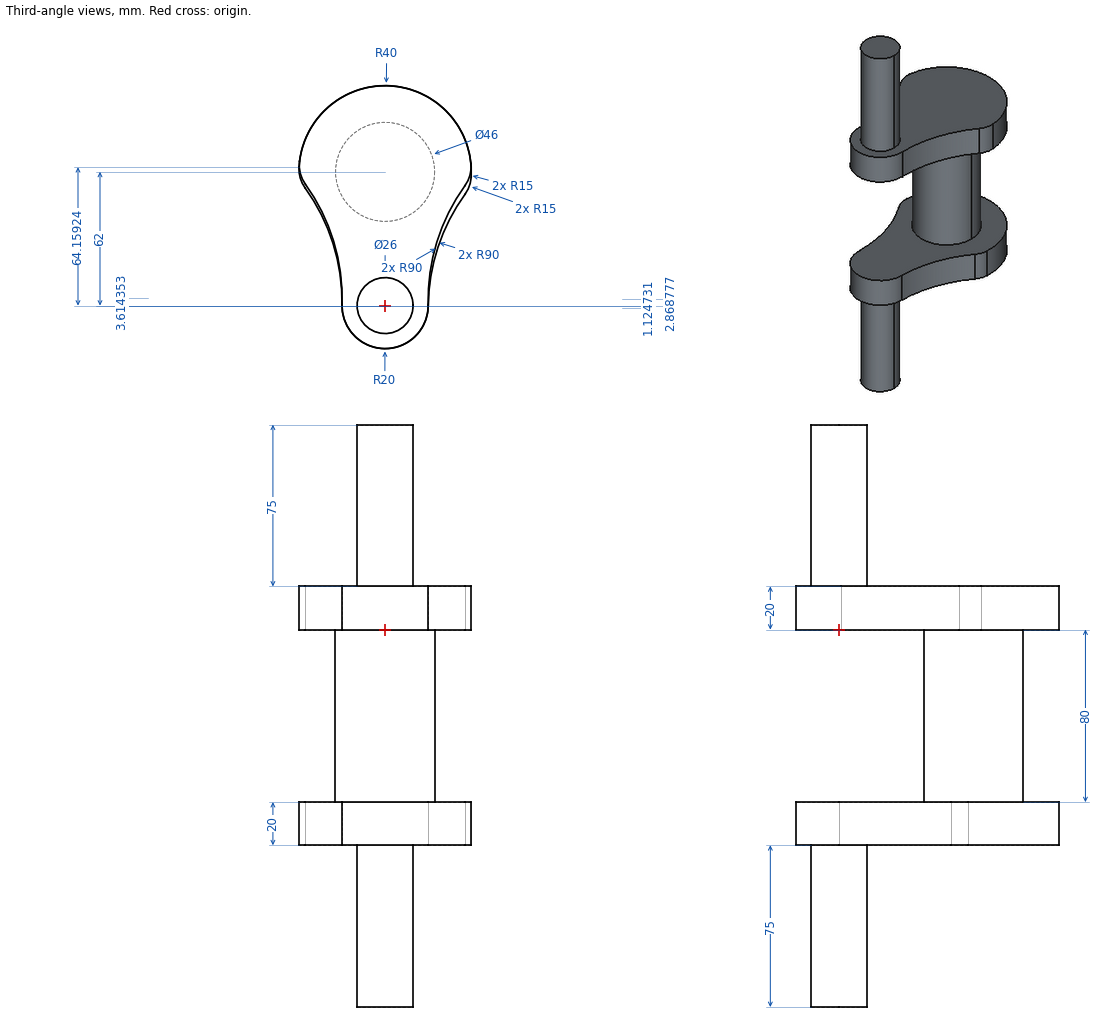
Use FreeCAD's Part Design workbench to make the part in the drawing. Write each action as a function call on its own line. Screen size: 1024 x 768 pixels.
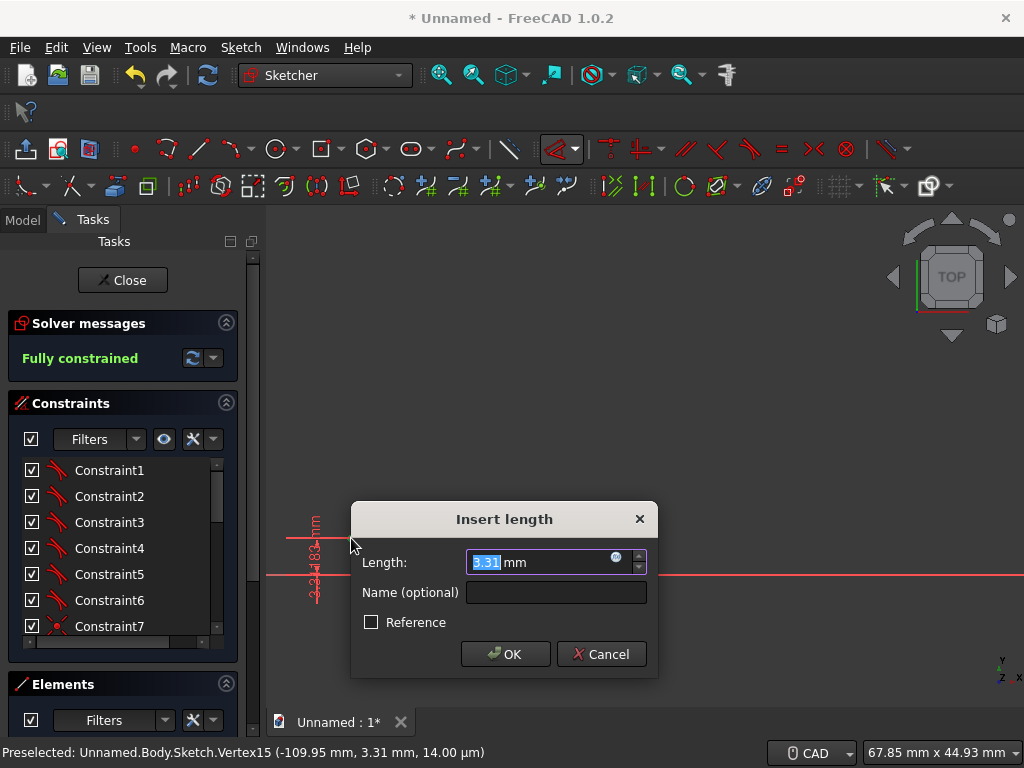
text(3.614353)
key(Return)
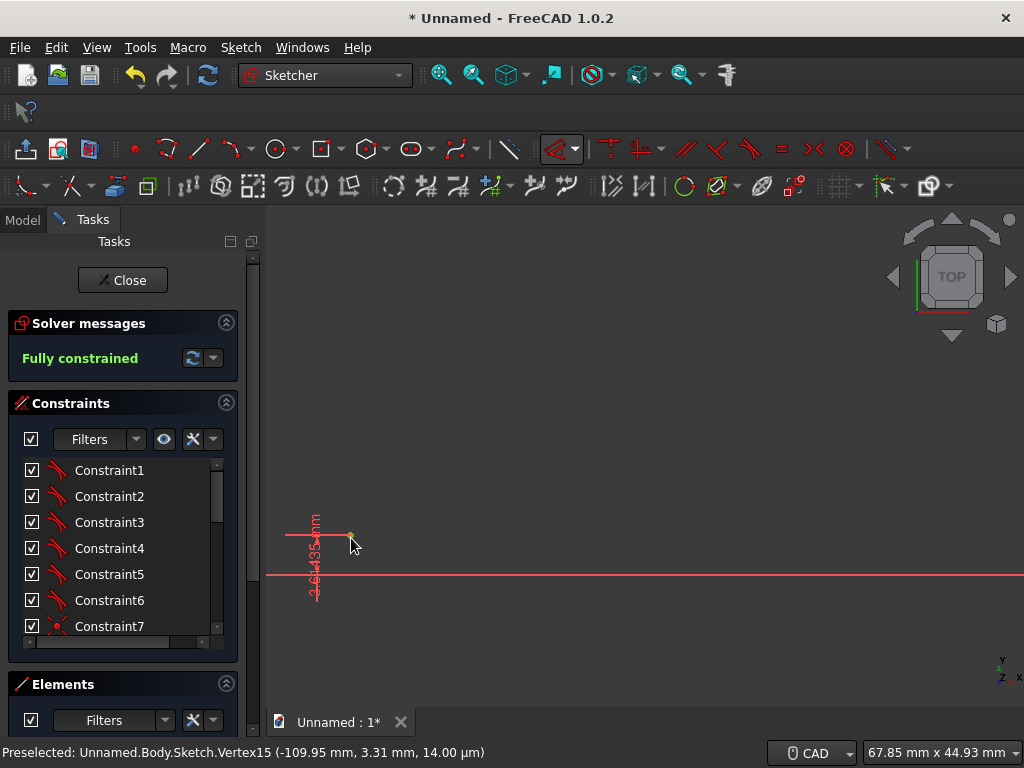
click(123, 280)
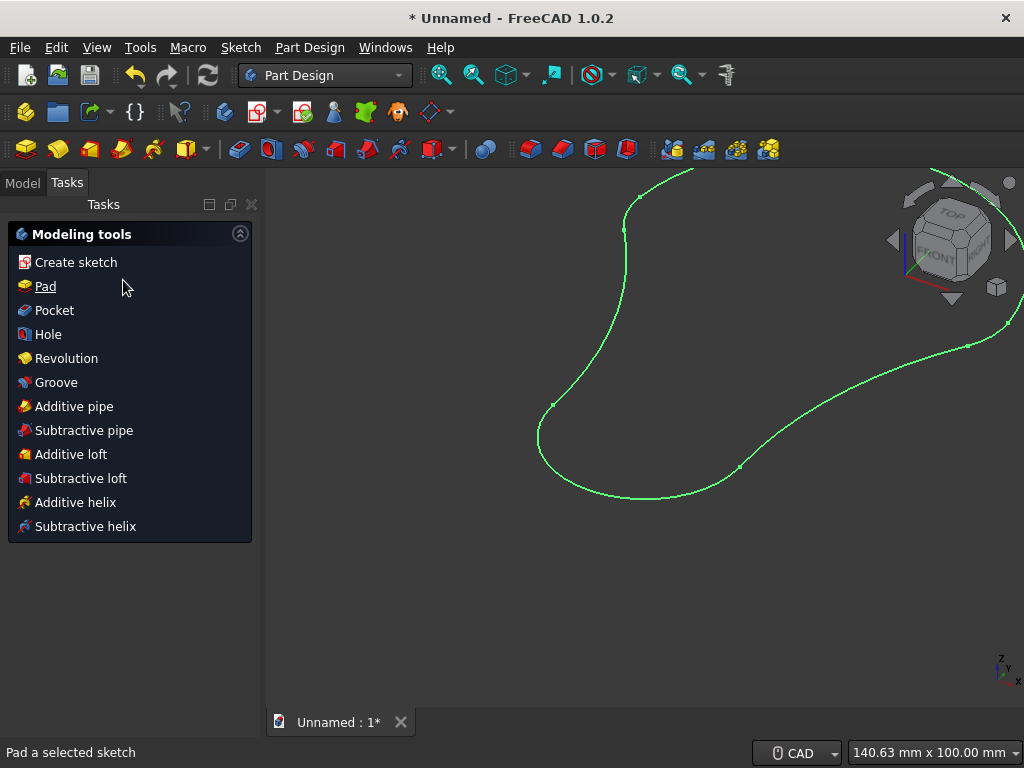
click(26, 150)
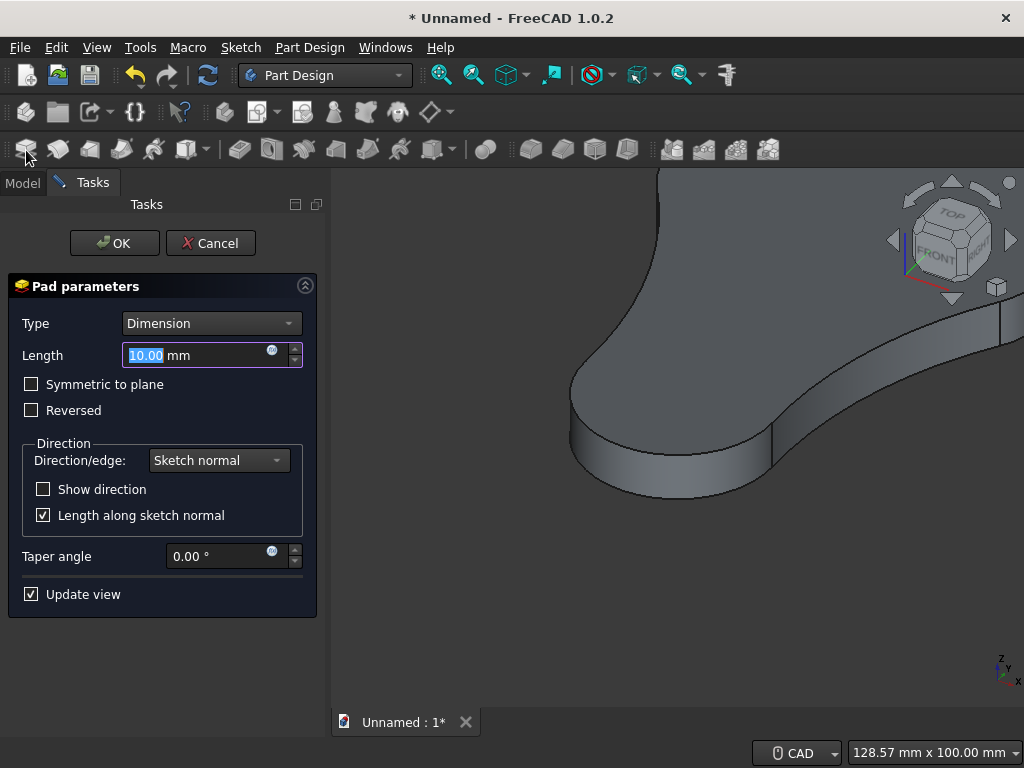
text(20)
key(Tab)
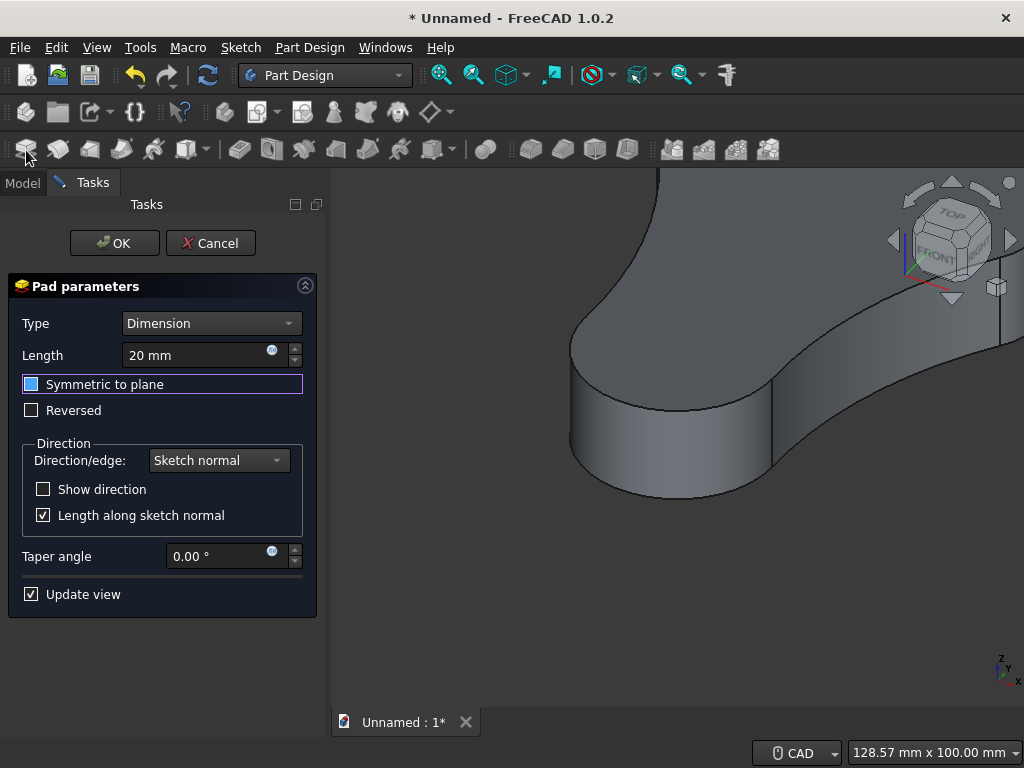
click(115, 243)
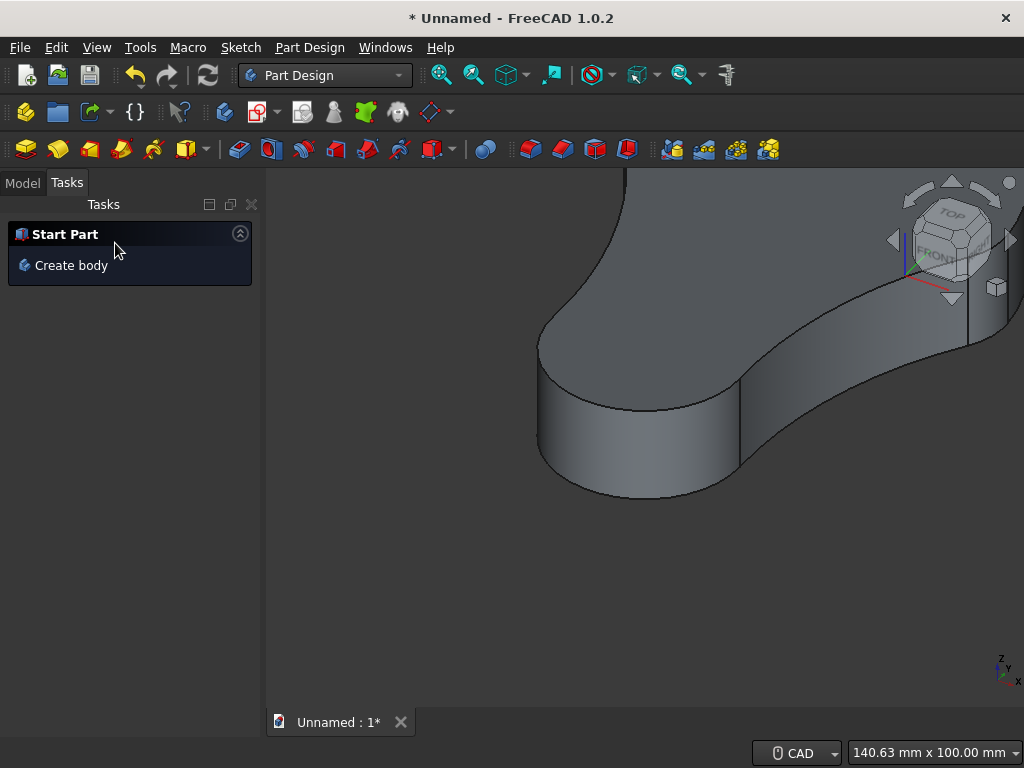
key(v)
key(f)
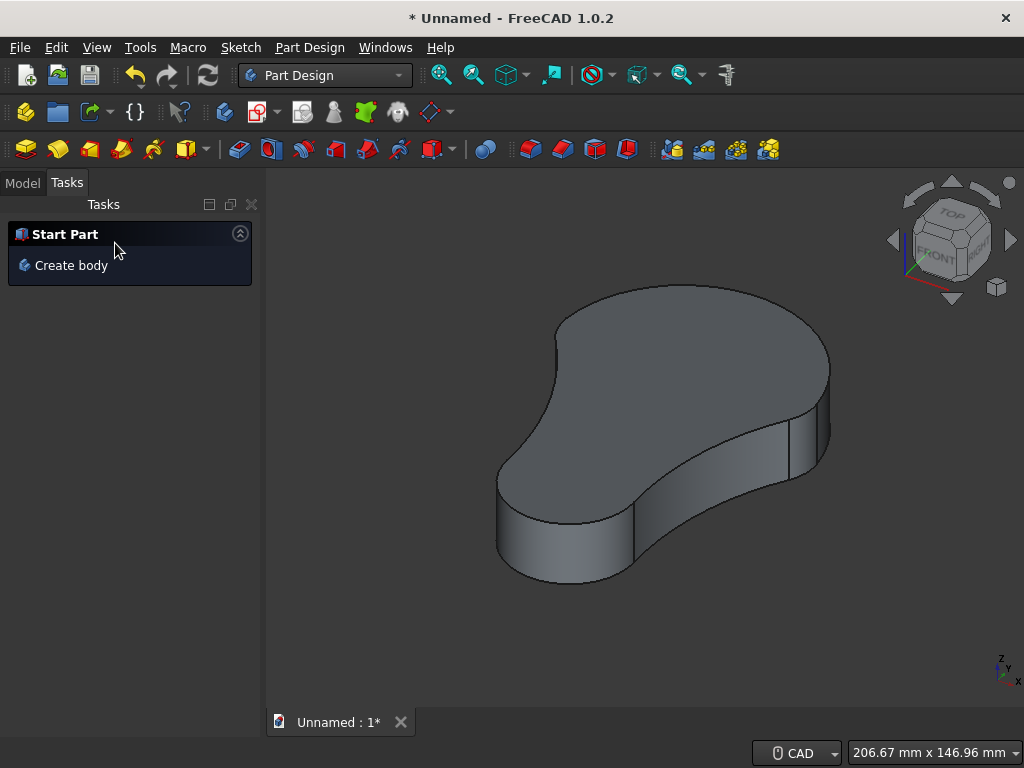
click(677, 375)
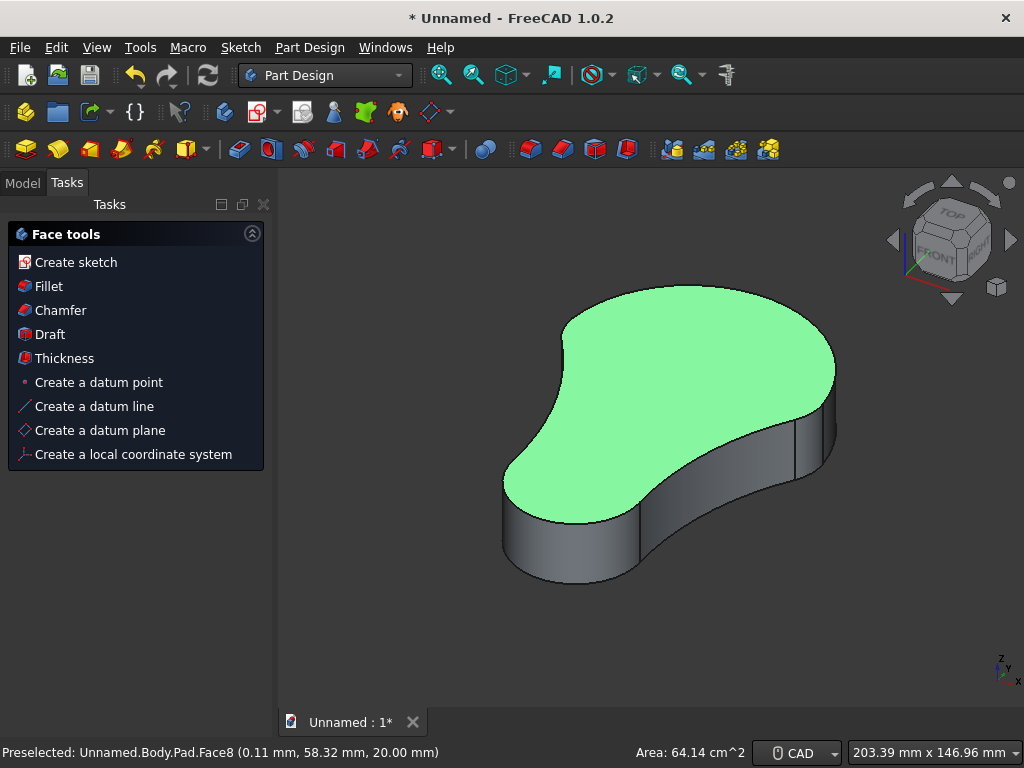
click(258, 112)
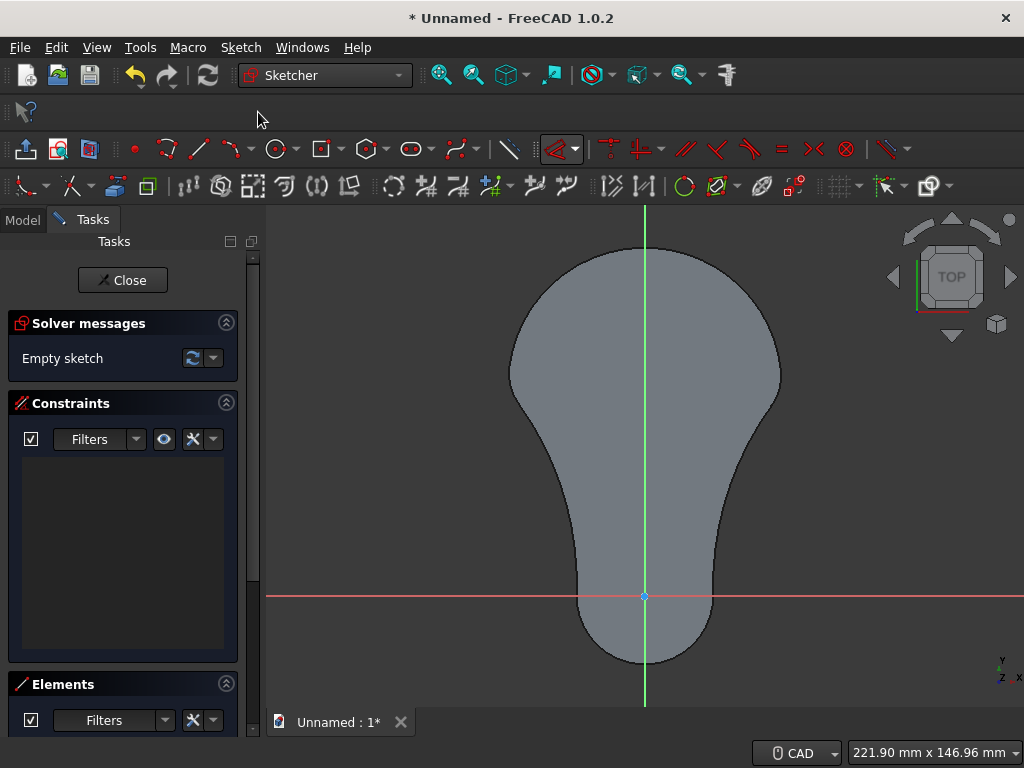
scroll(674, 656, up, 6)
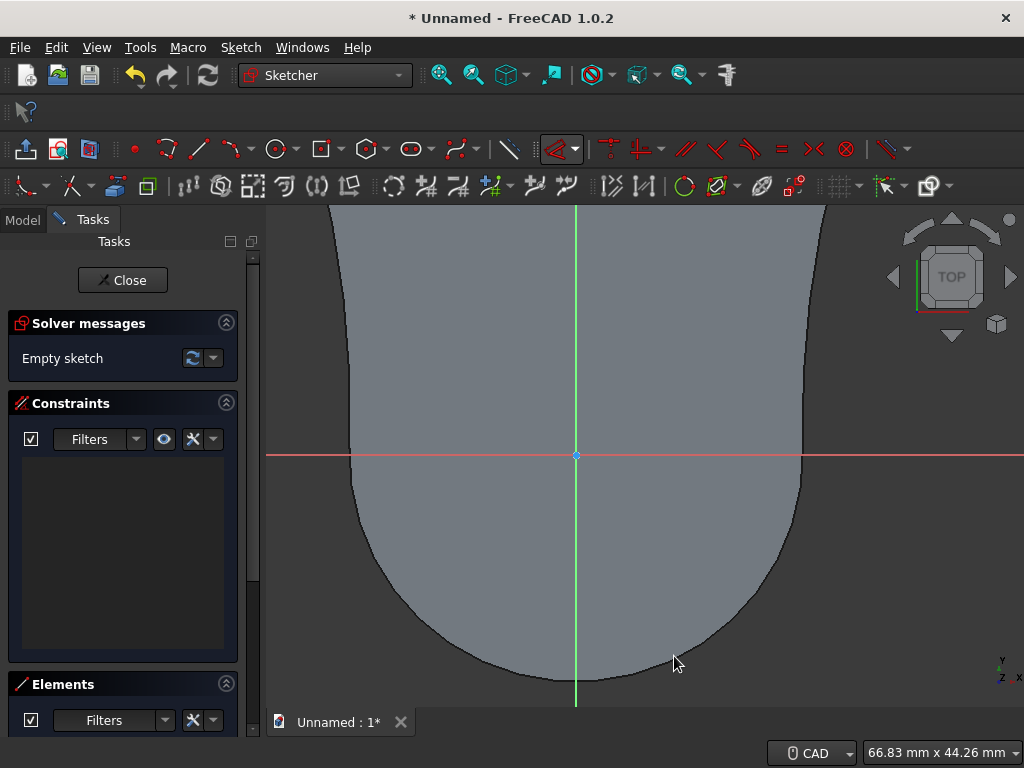
key(g)
key(c)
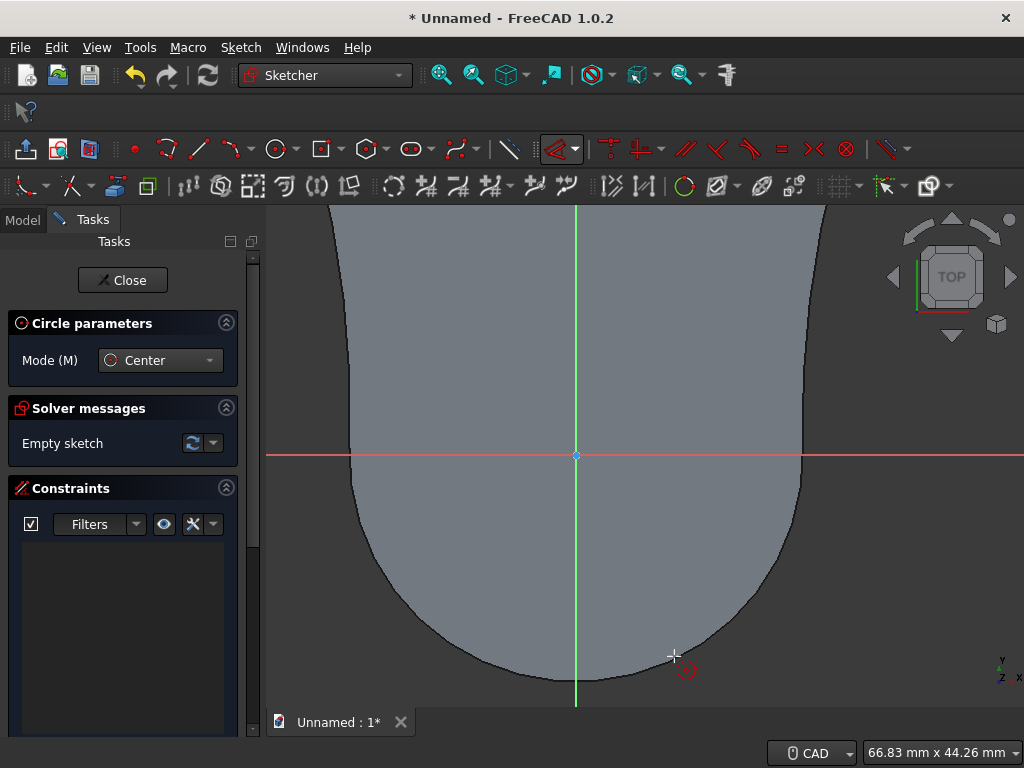
click(576, 455)
move(680, 351)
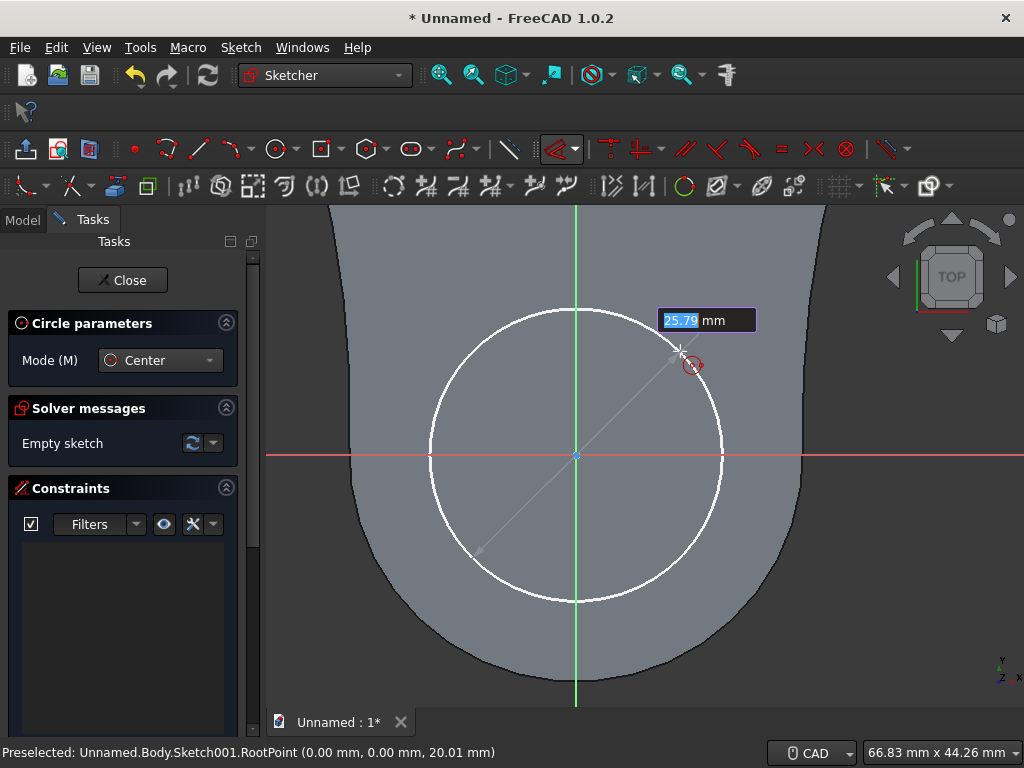
text(26)
key(Return)
key(Escape)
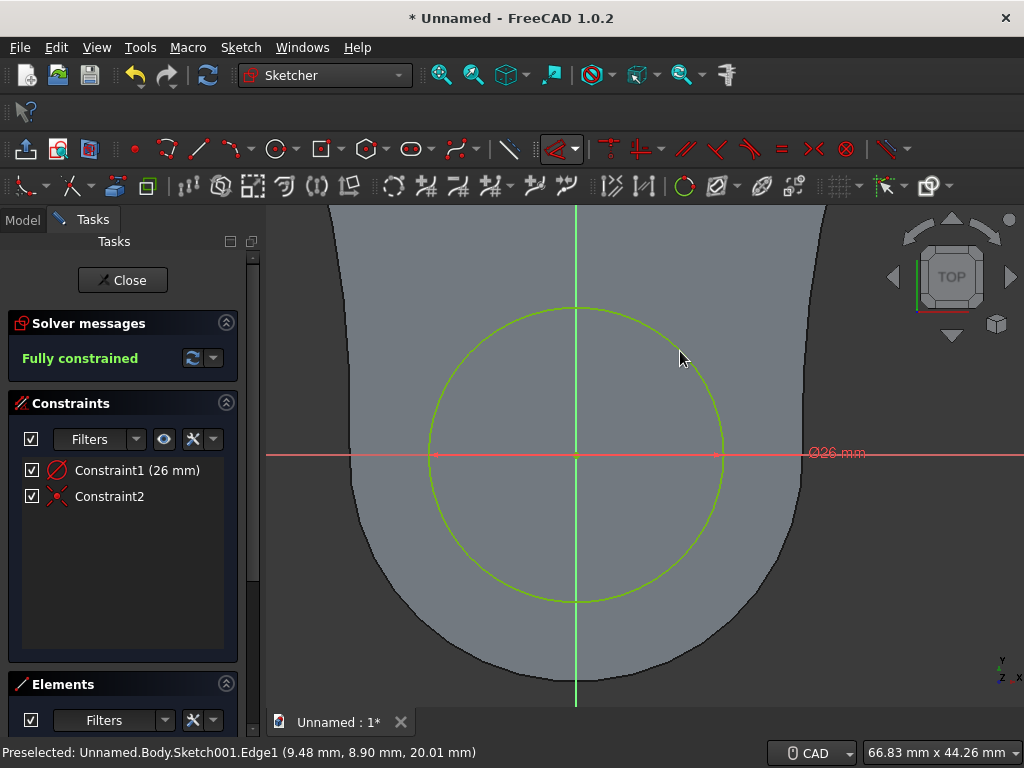
click(123, 280)